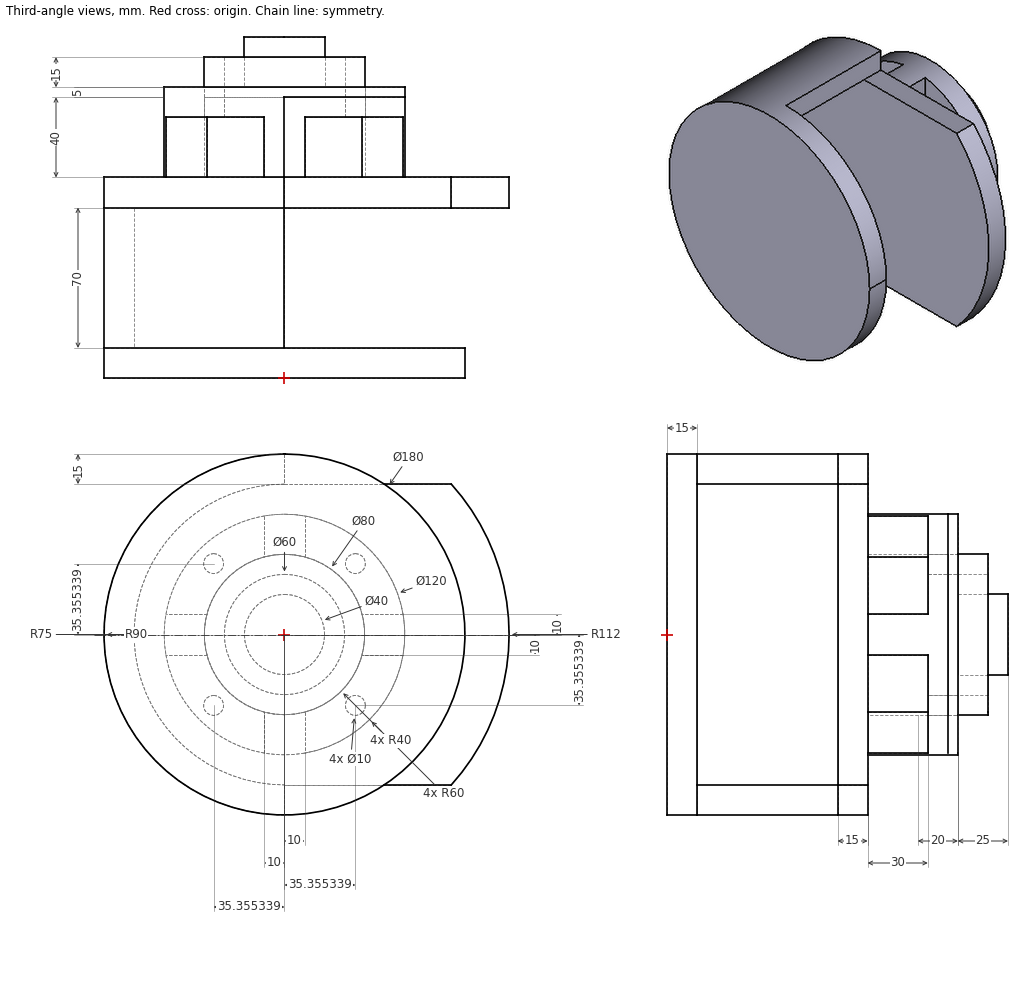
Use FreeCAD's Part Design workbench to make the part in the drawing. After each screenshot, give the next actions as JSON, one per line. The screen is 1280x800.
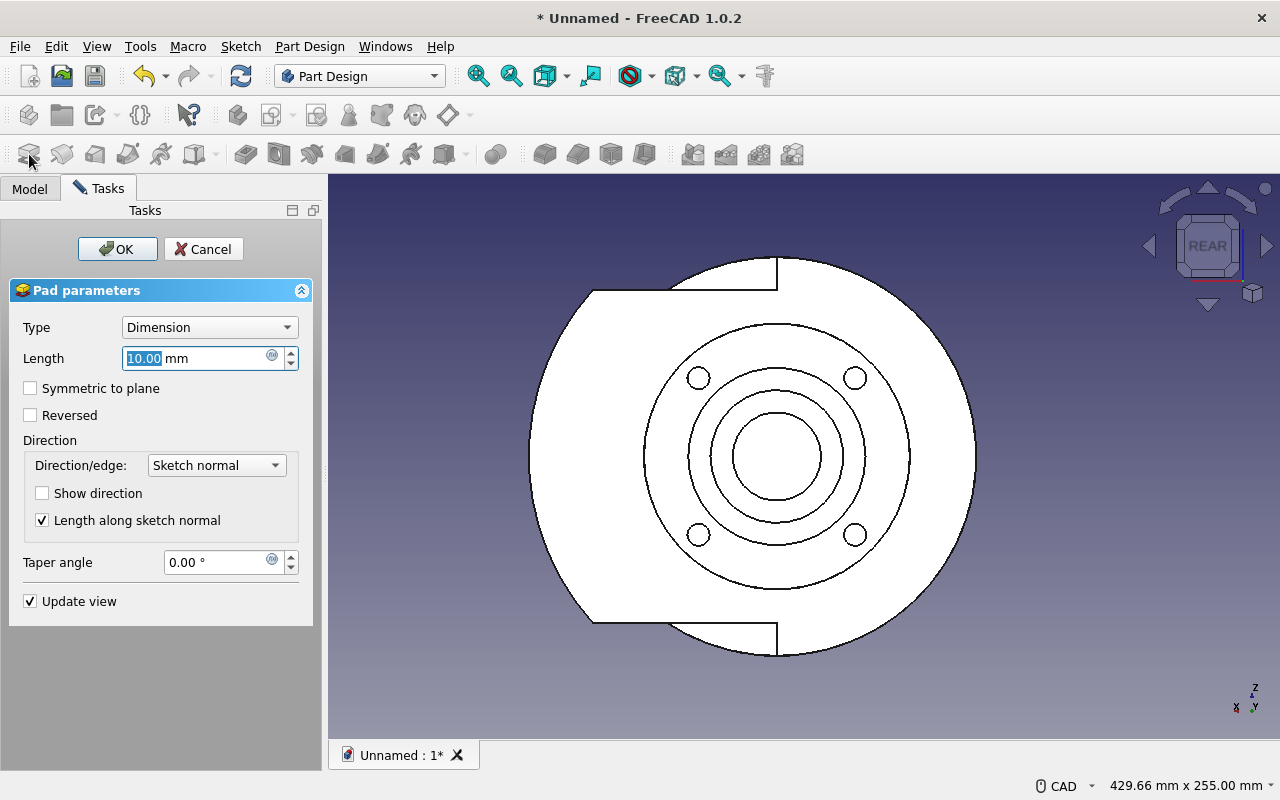
{"action": "type", "text": "25"}
{"action": "key", "text": "Tab"}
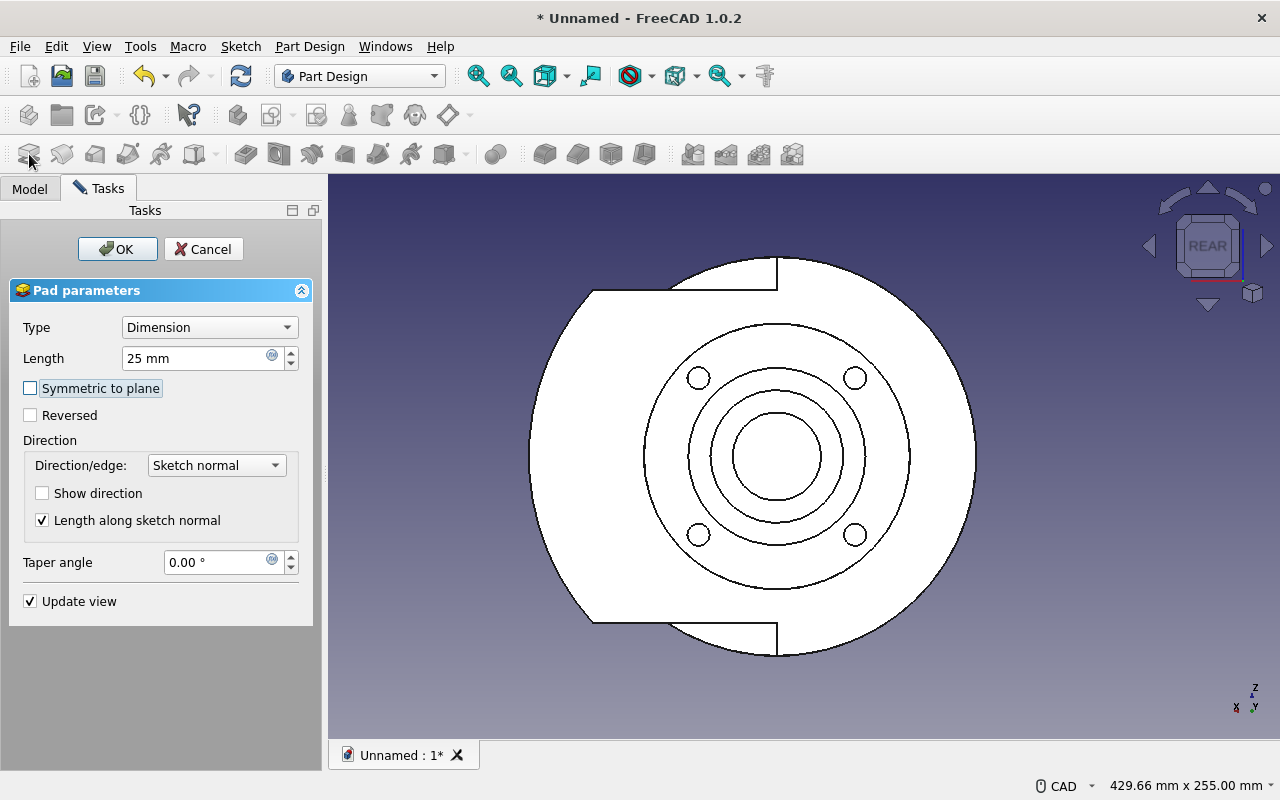
{"action": "left_click", "coordinate": [118, 249]}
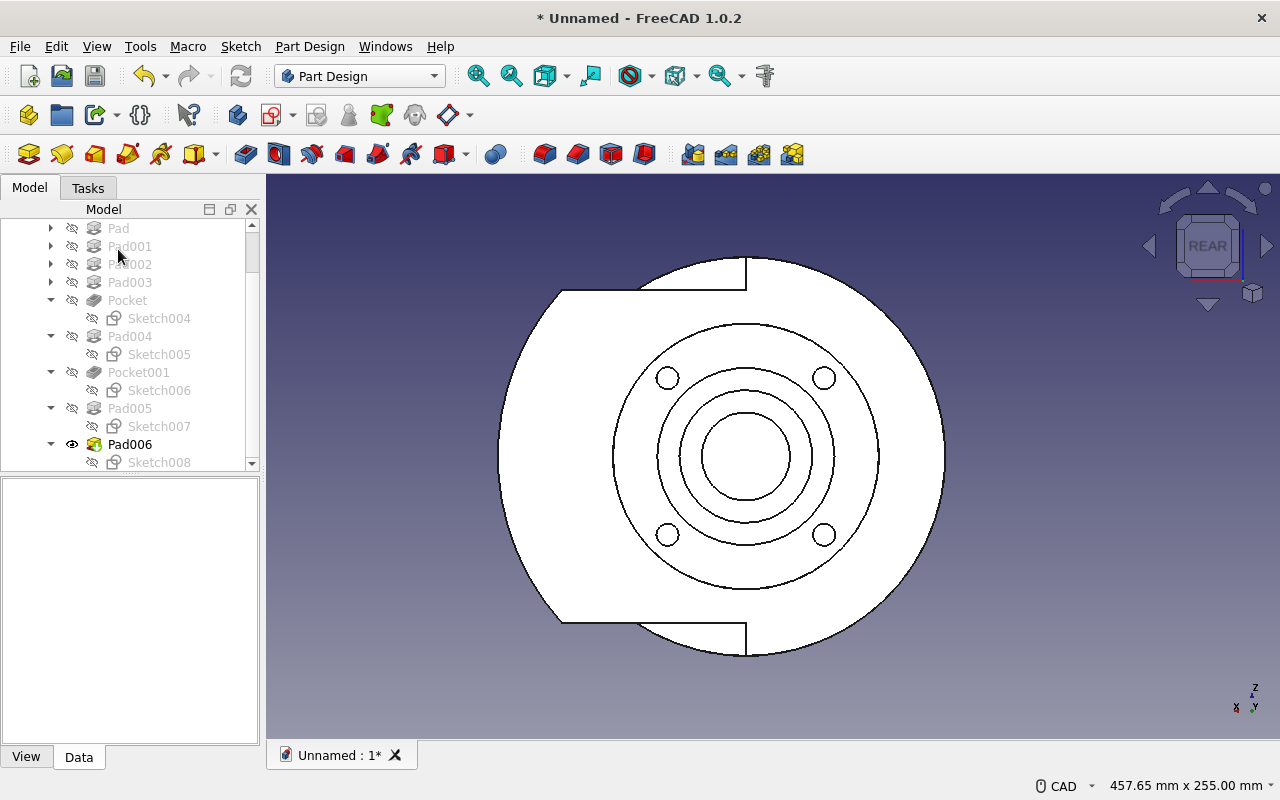
{"action": "key", "text": "0"}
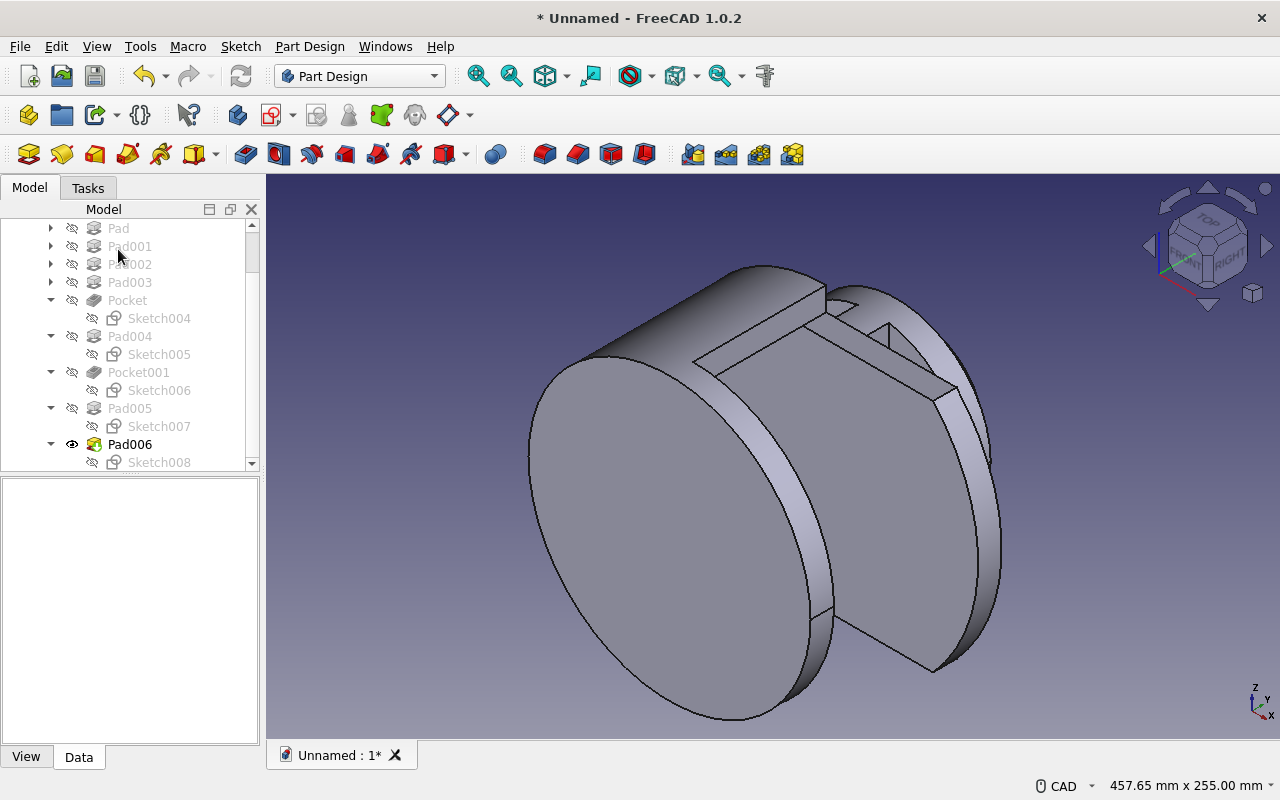
{"action": "left_click", "coordinate": [479, 76]}